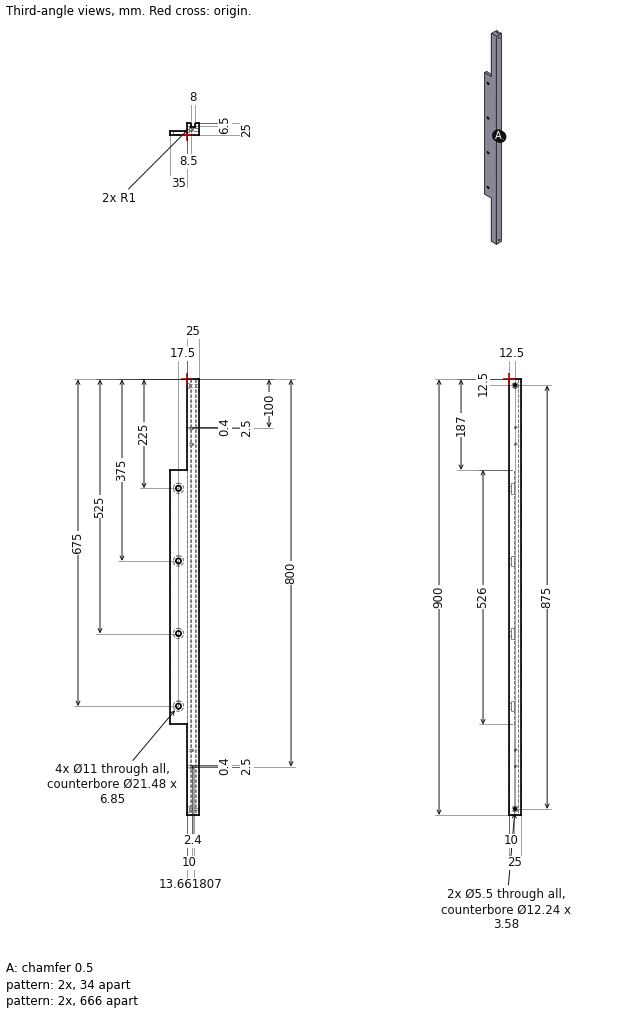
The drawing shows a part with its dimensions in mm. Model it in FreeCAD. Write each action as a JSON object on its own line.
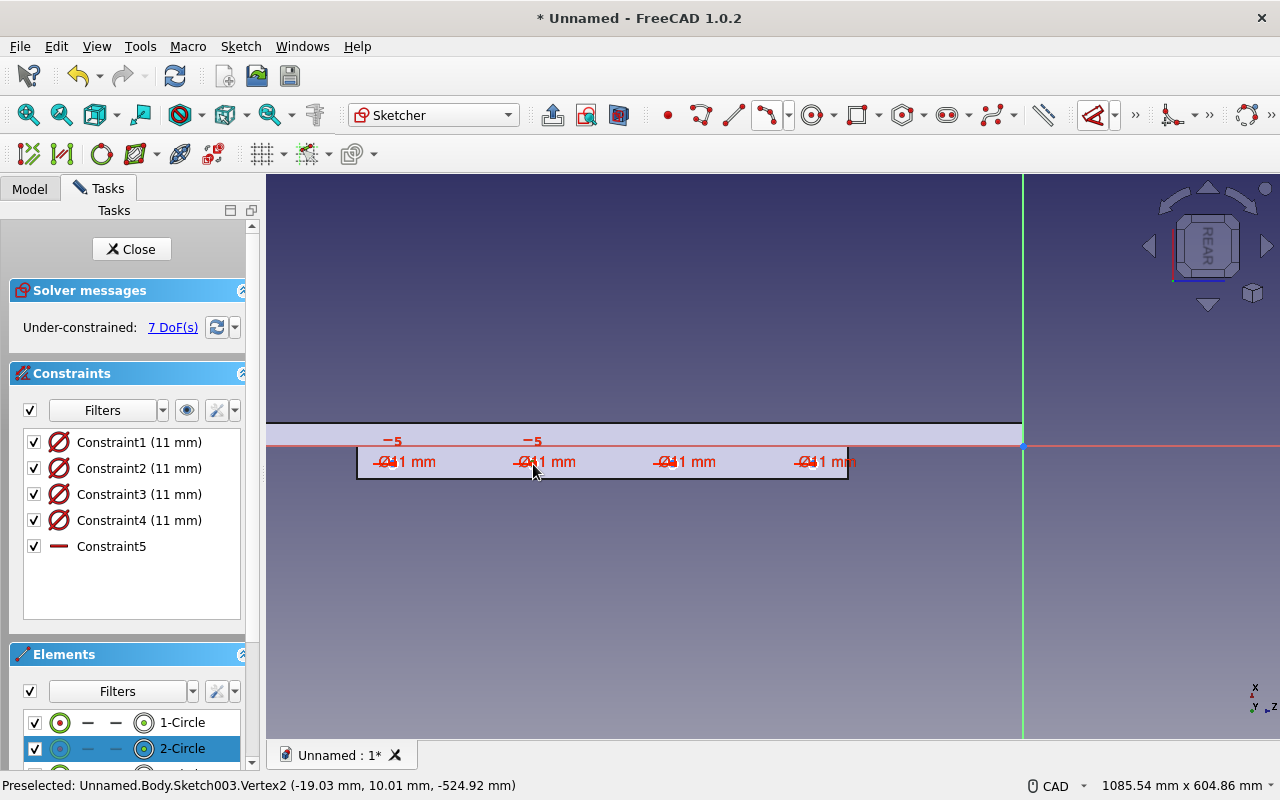
{"action": "left_click", "coordinate": [673, 464]}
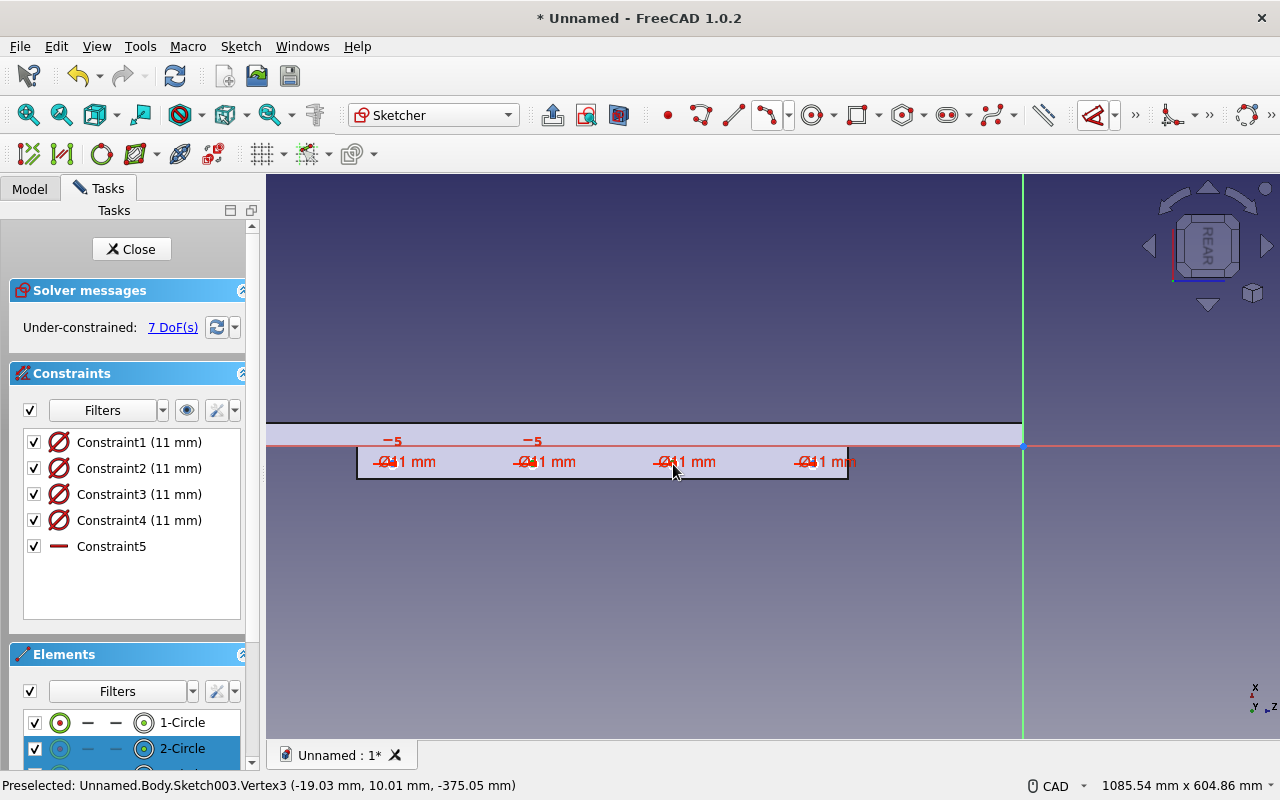
{"action": "key", "text": "h"}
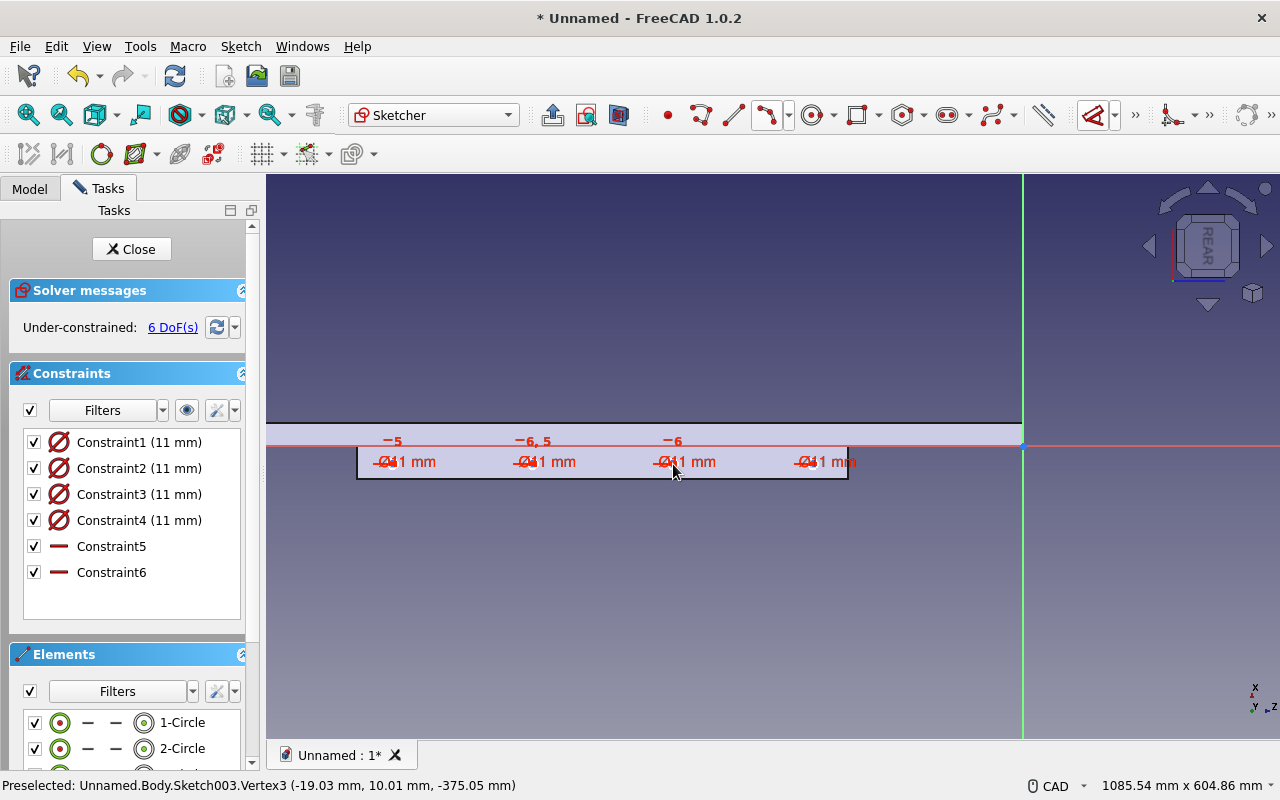
{"action": "left_click", "coordinate": [673, 464]}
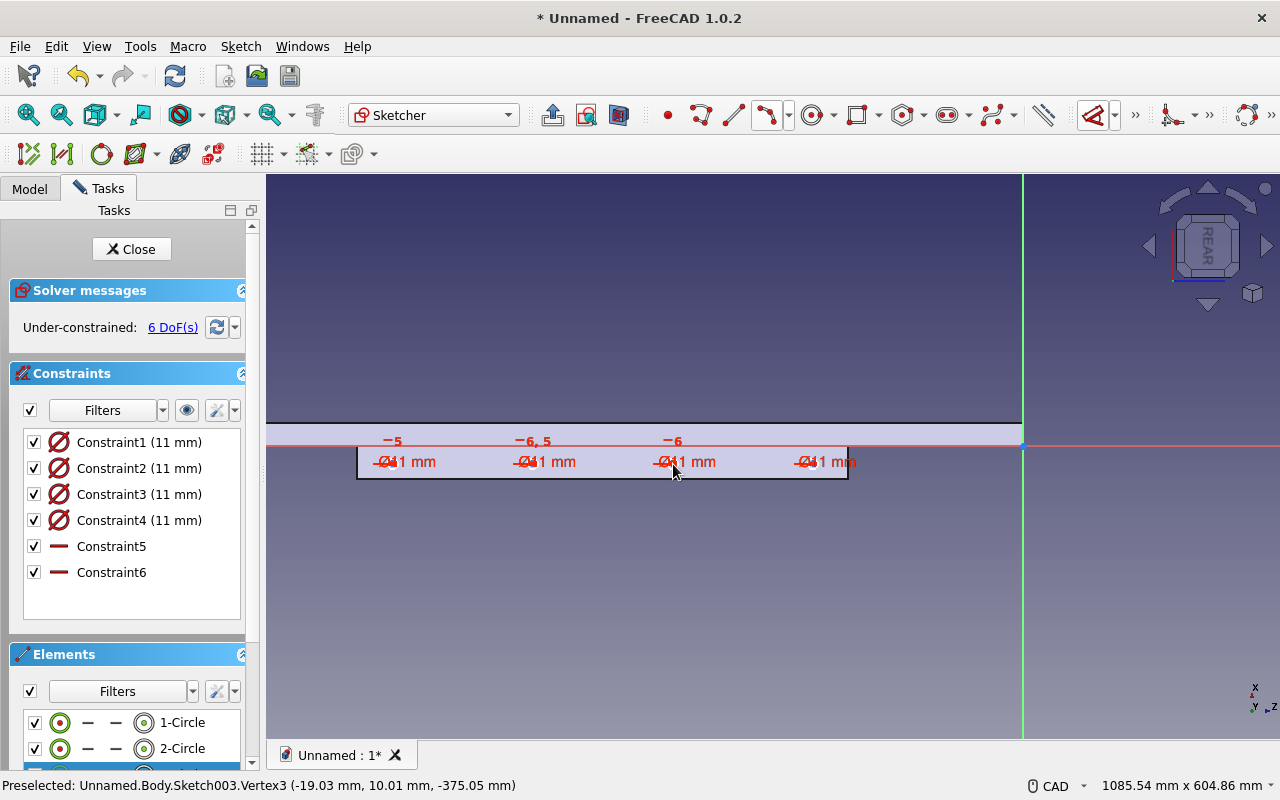
{"action": "left_click", "coordinate": [813, 464]}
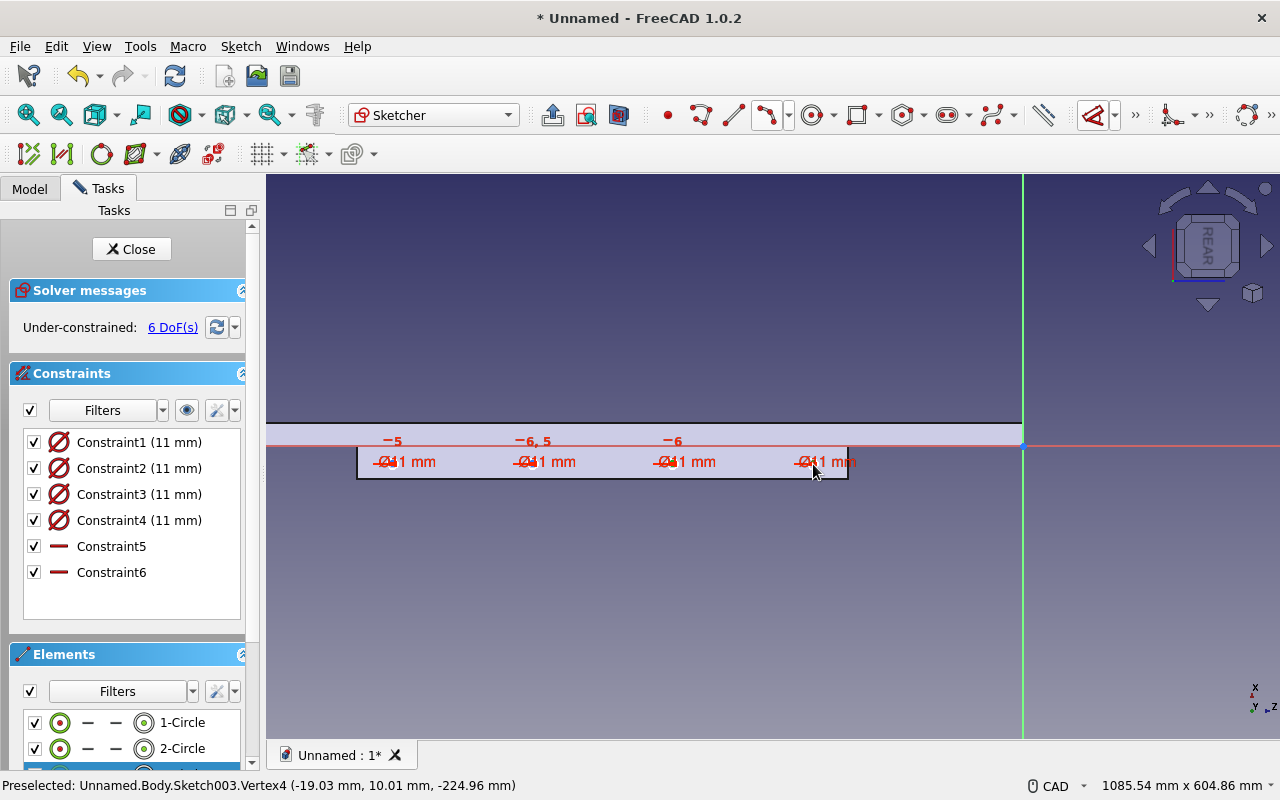
{"action": "key", "text": "h"}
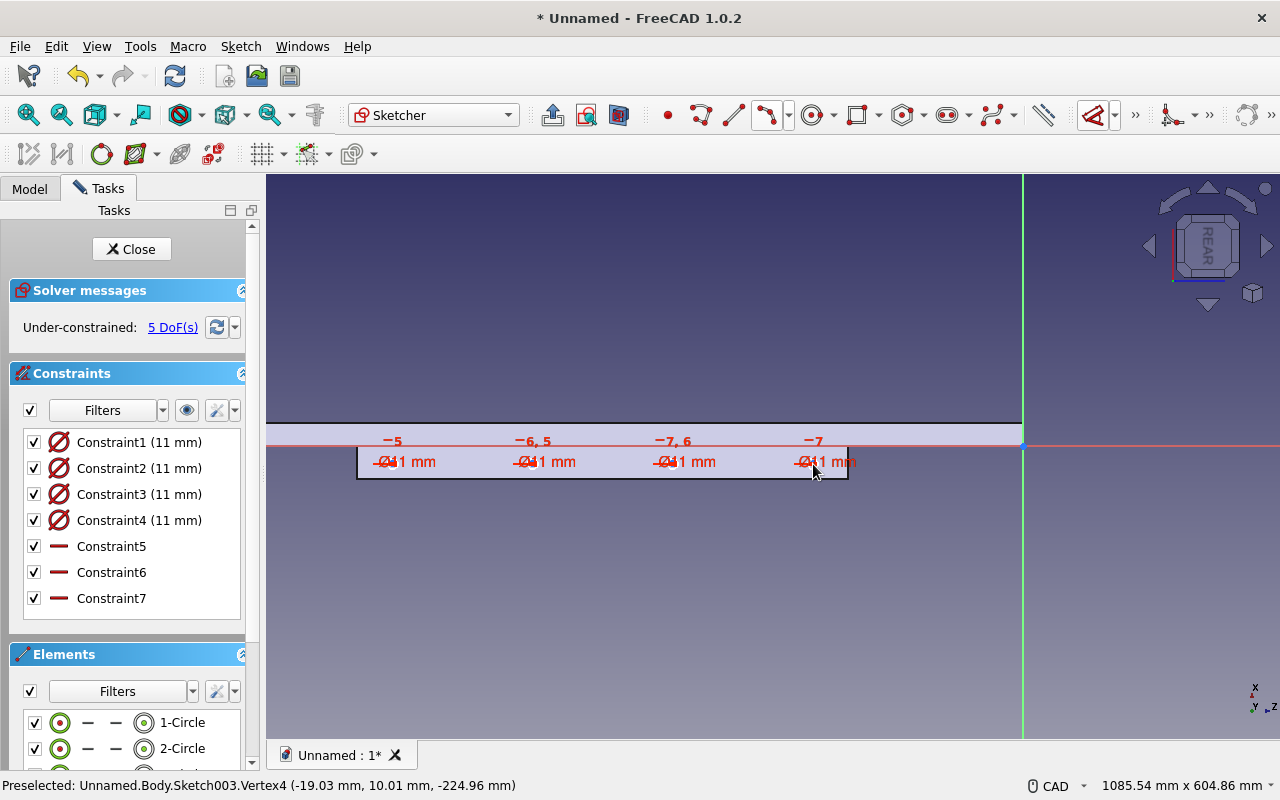
{"action": "left_click", "coordinate": [393, 464]}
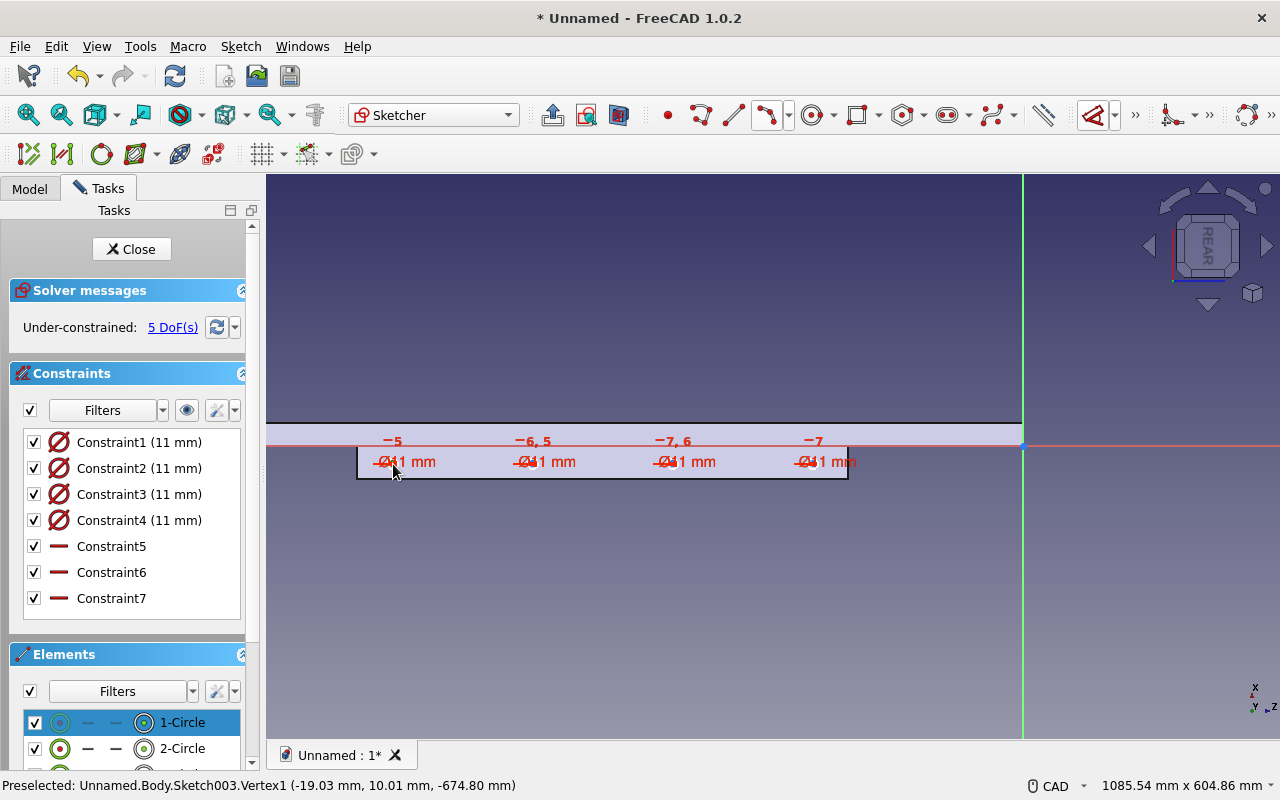
{"action": "key", "text": "l"}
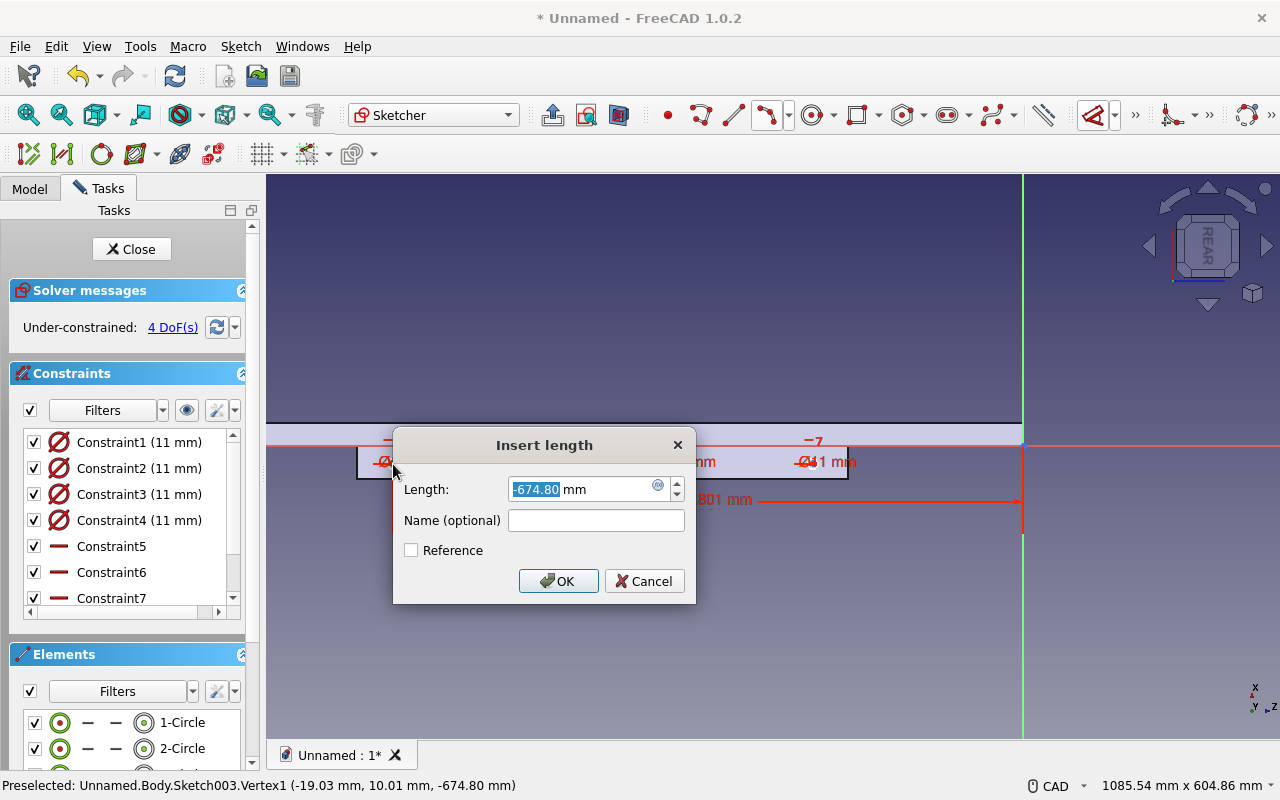
{"action": "type", "text": "-675"}
{"action": "key", "text": "Return"}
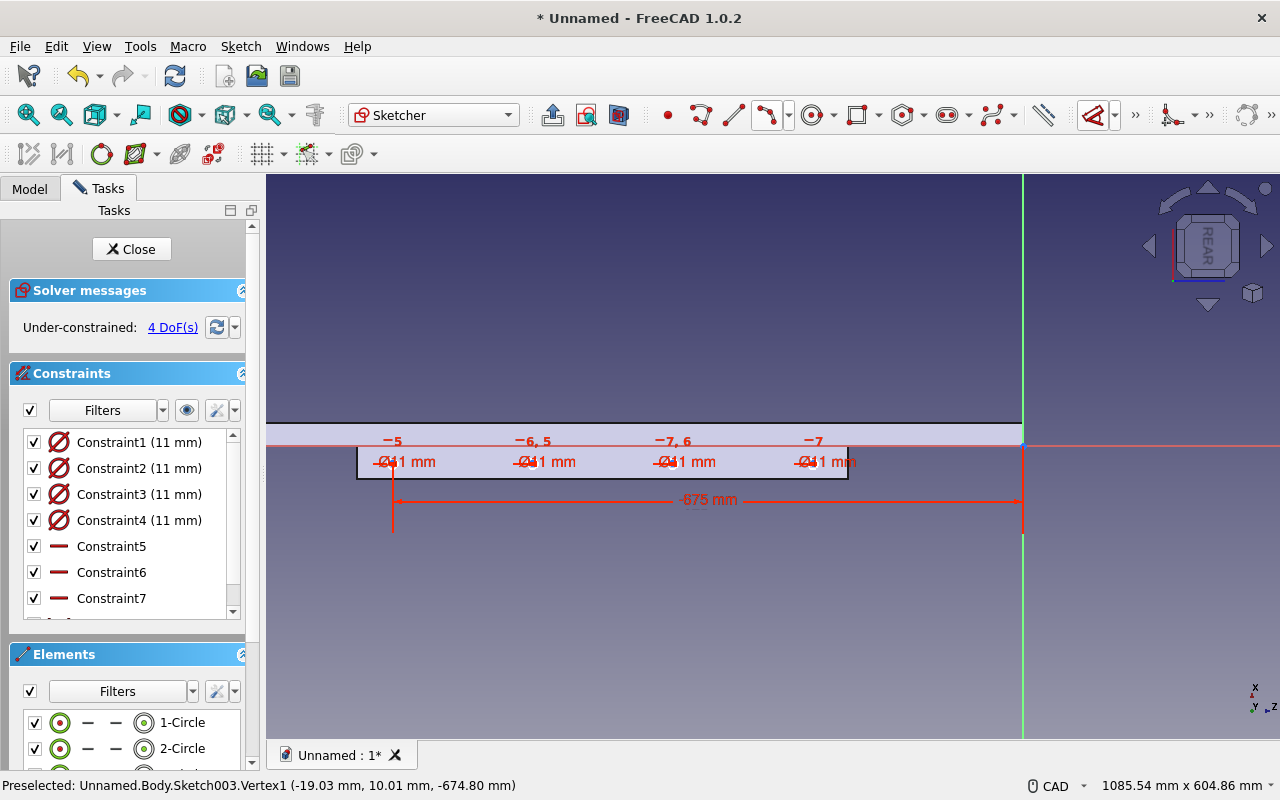
{"action": "left_click", "coordinate": [533, 464]}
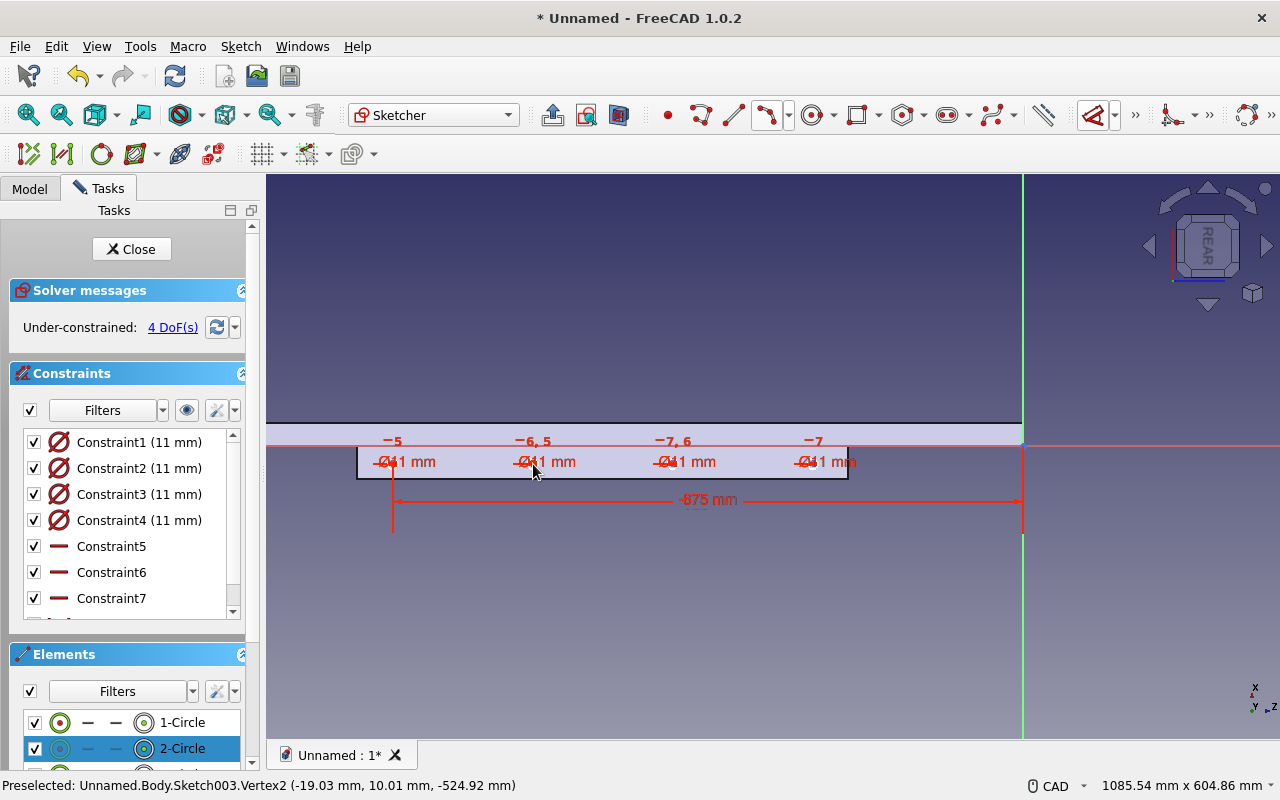
{"action": "left_click", "coordinate": [1114, 116]}